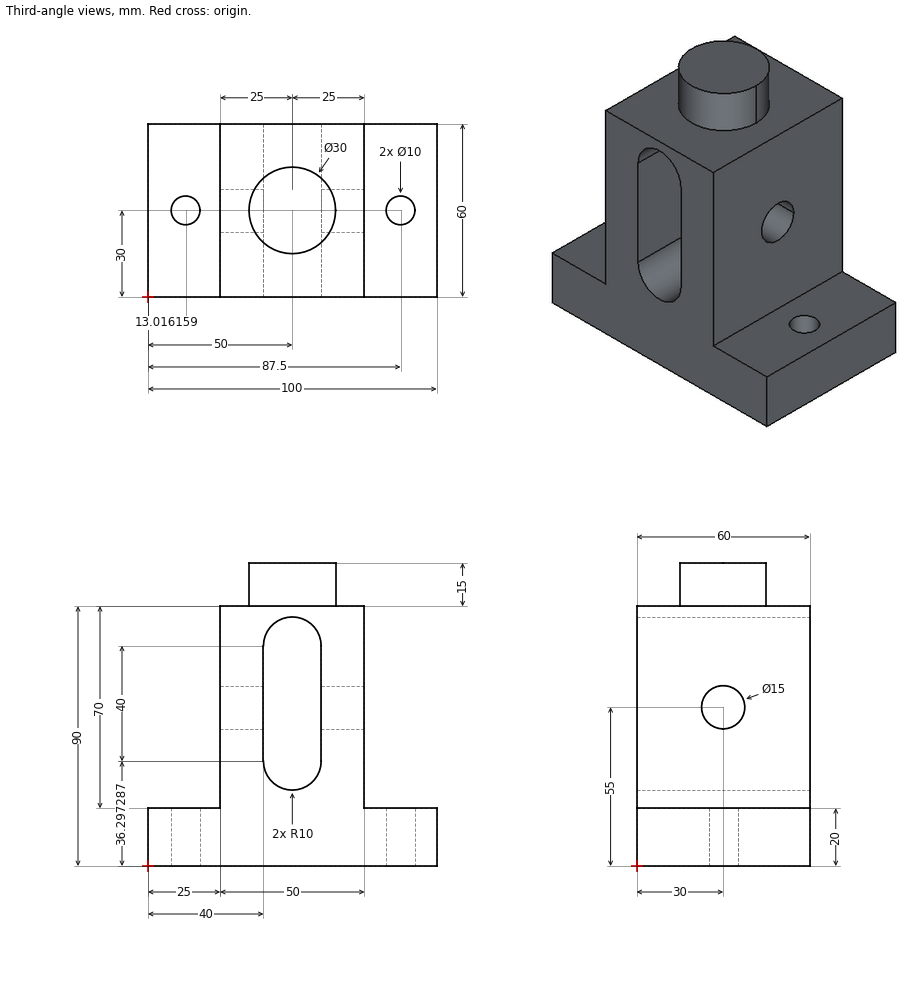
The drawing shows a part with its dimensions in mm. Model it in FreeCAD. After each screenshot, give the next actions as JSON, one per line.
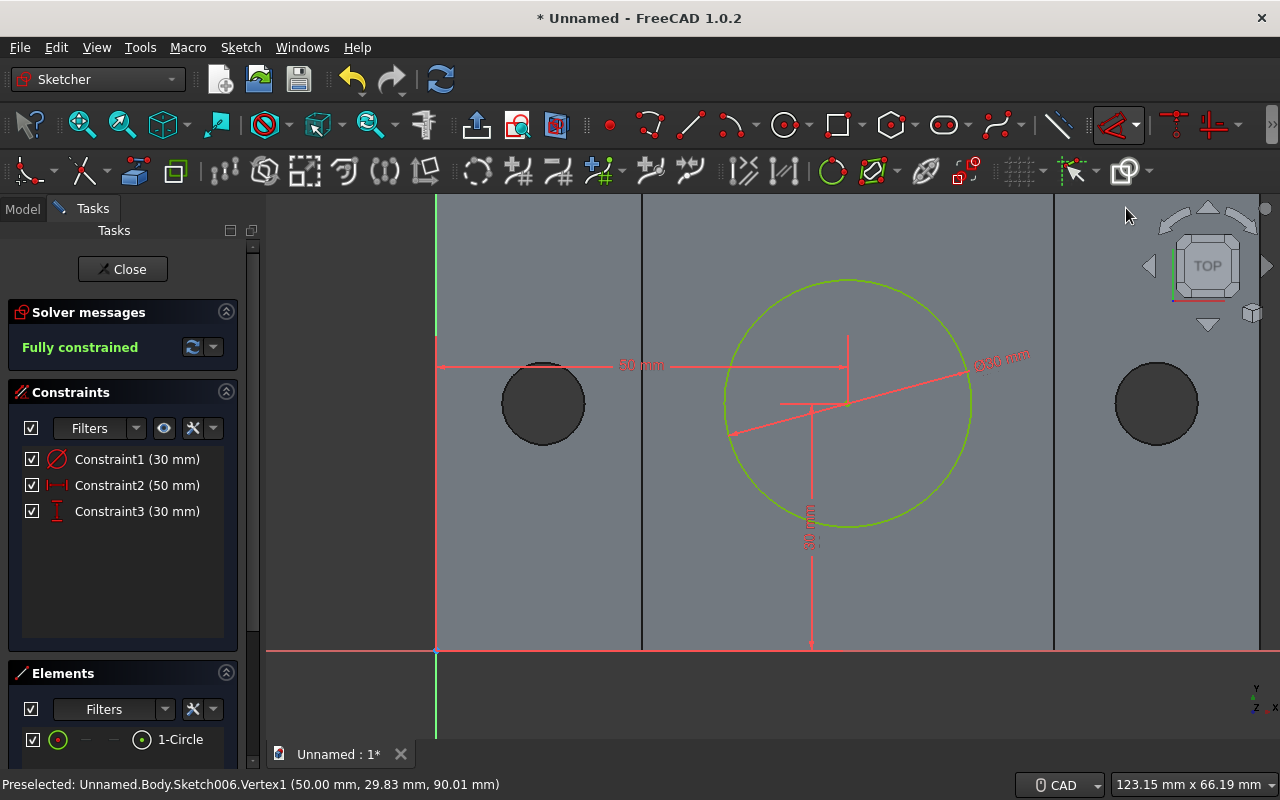
{"action": "left_click", "coordinate": [123, 269]}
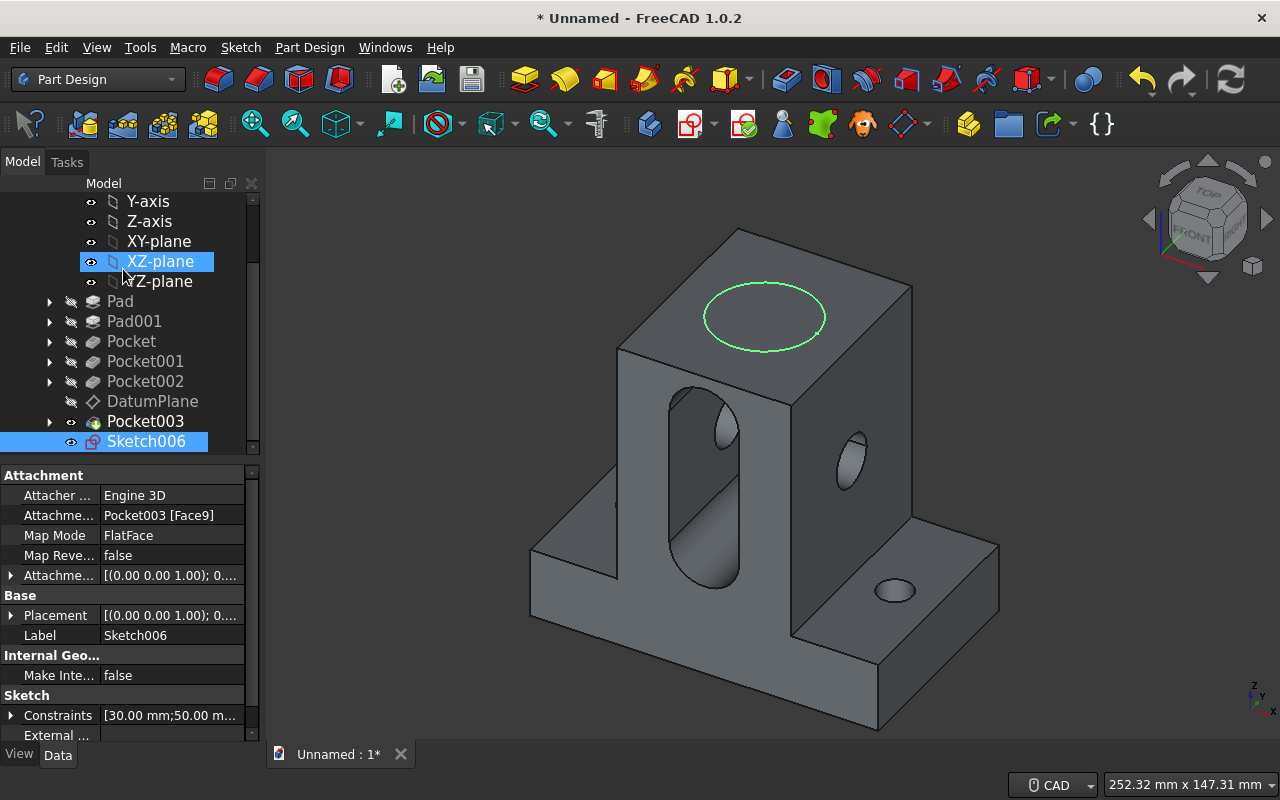
{"action": "left_click", "coordinate": [526, 80]}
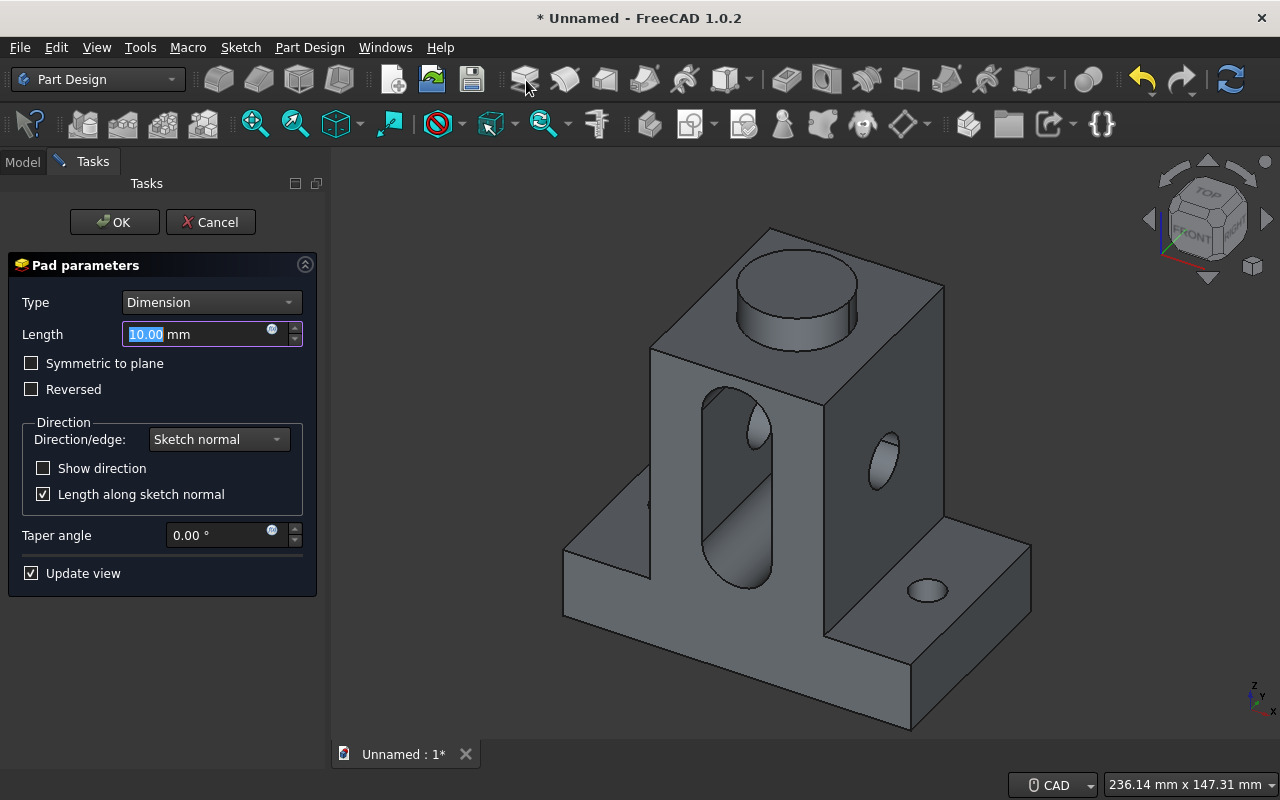
{"action": "type", "text": "15"}
{"action": "key", "text": "Tab"}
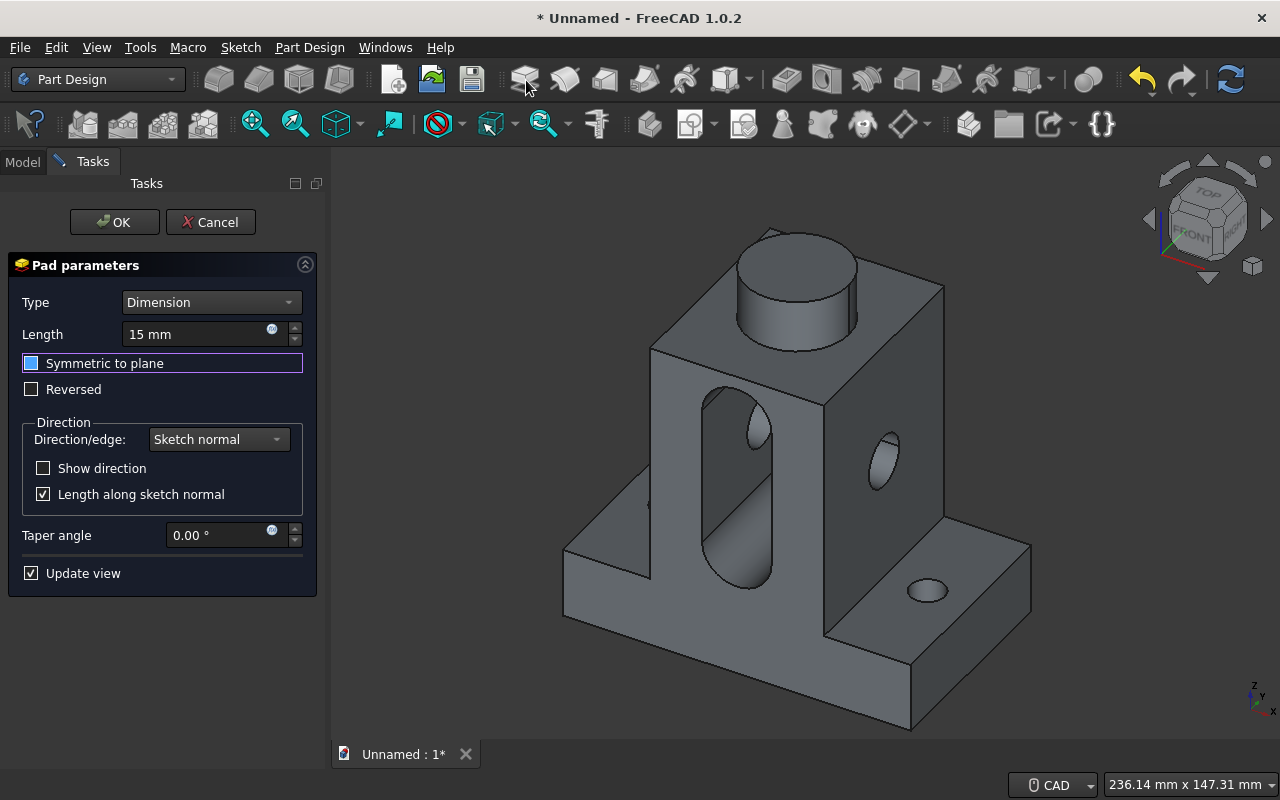
{"action": "left_click", "coordinate": [115, 222]}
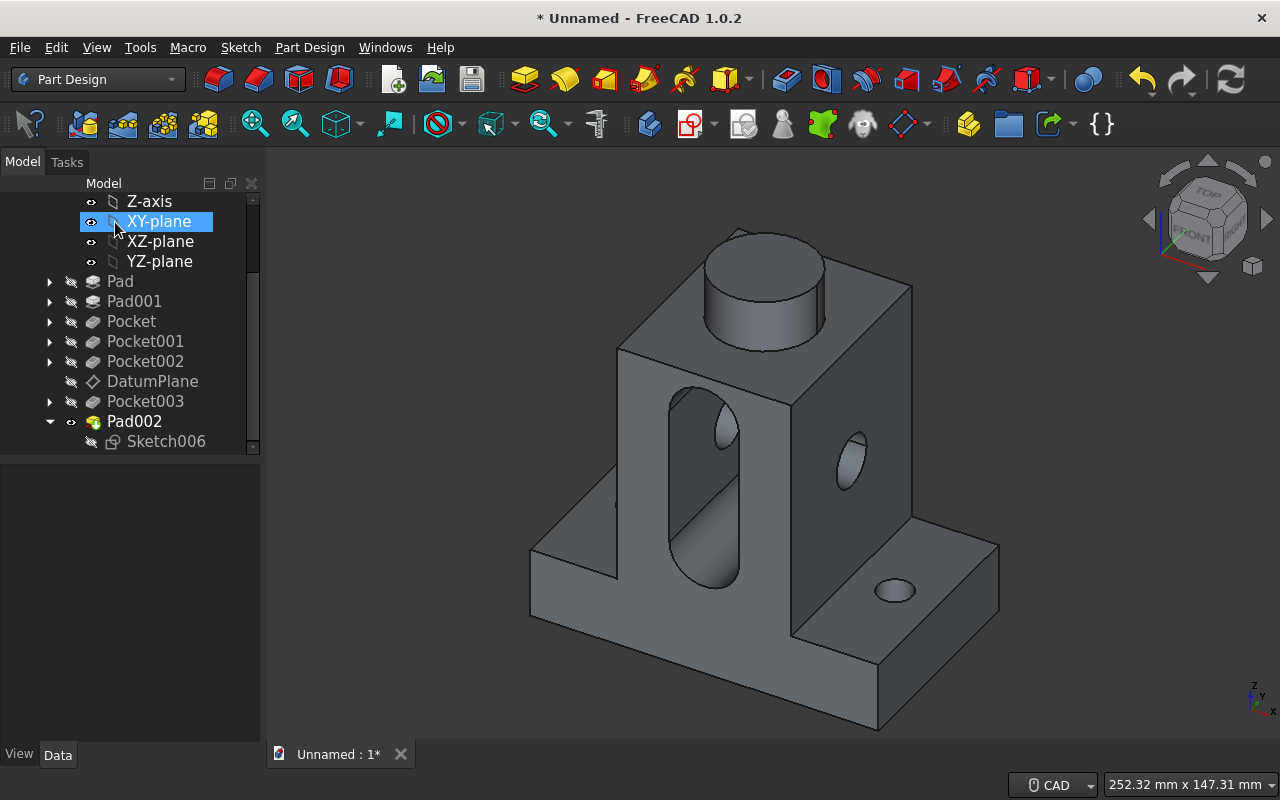
{"action": "key", "text": "0"}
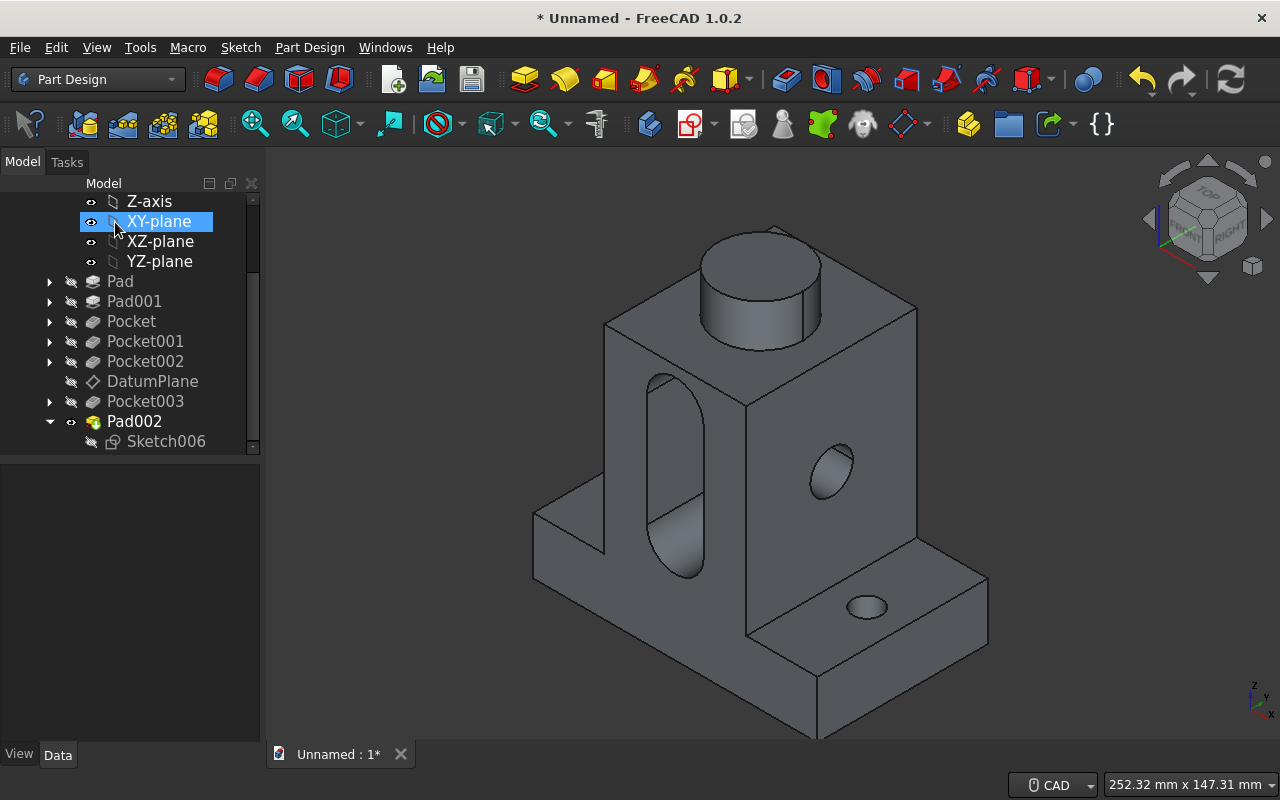
{"action": "left_click", "coordinate": [256, 124]}